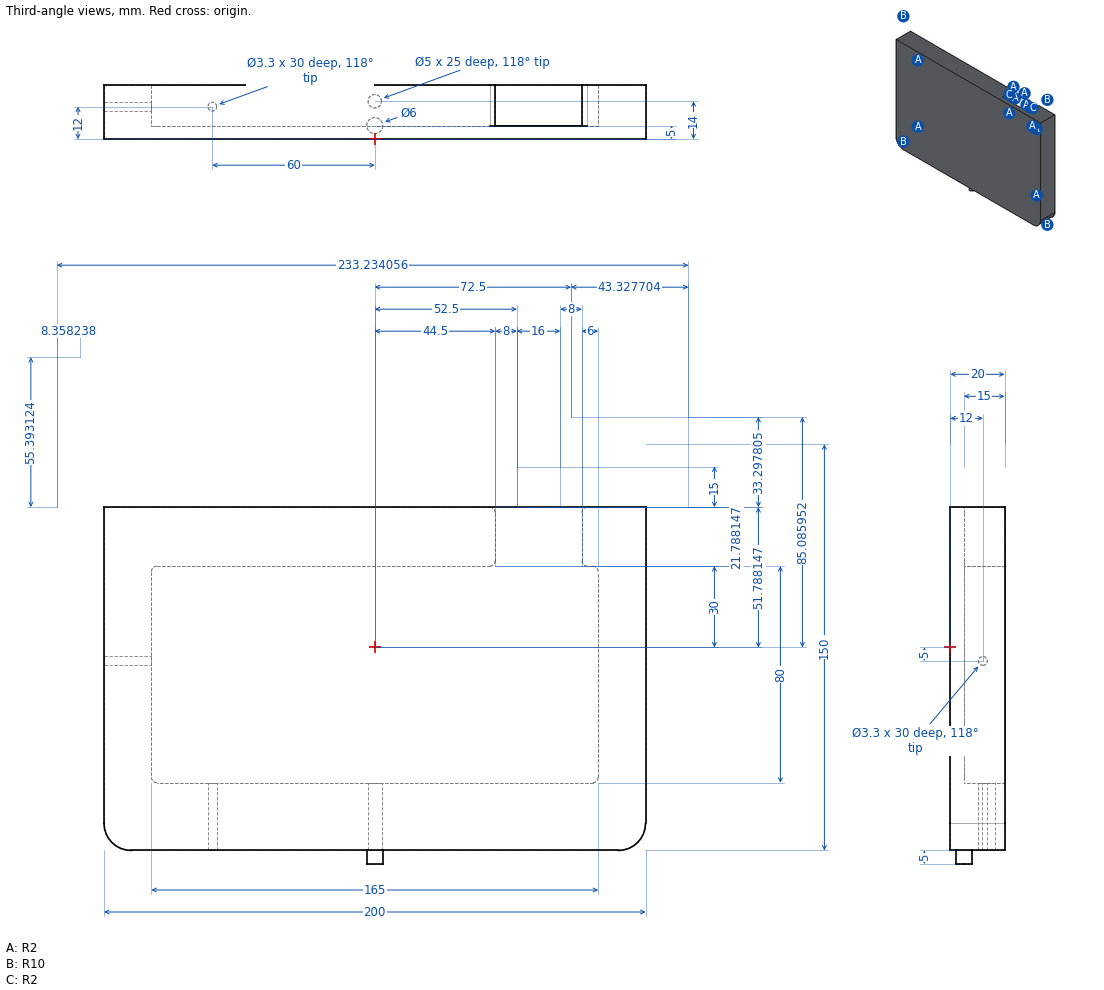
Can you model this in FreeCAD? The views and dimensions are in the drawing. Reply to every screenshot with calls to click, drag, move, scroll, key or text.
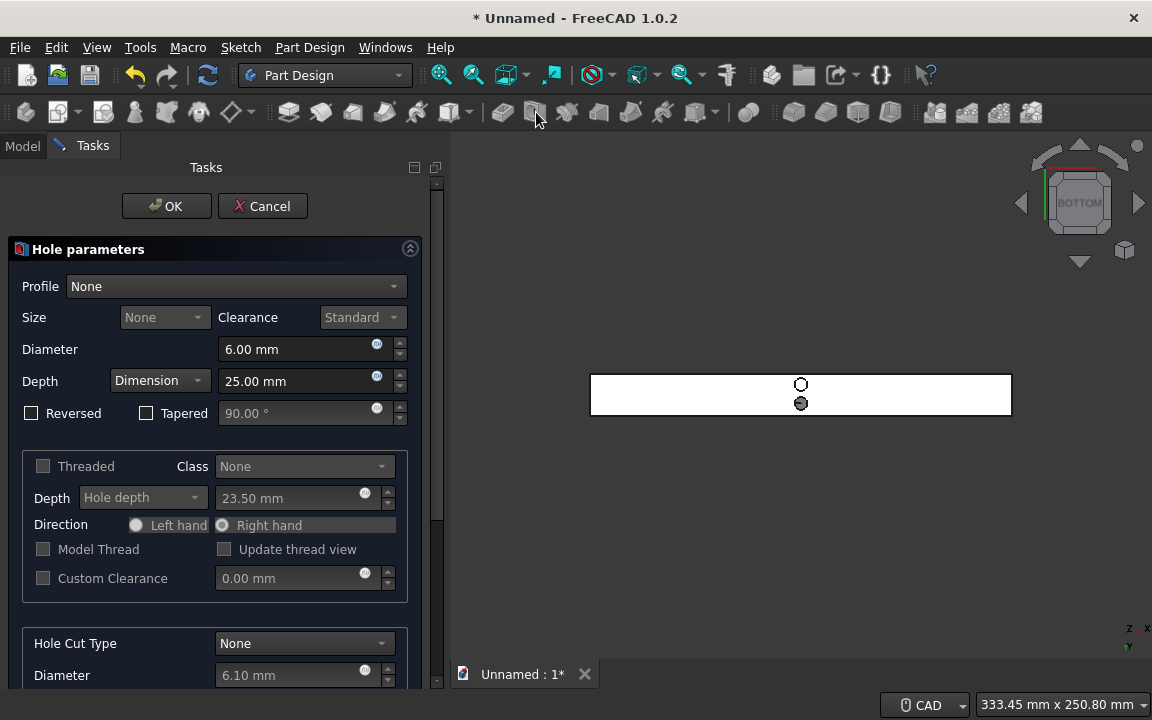
triple_click(305, 349)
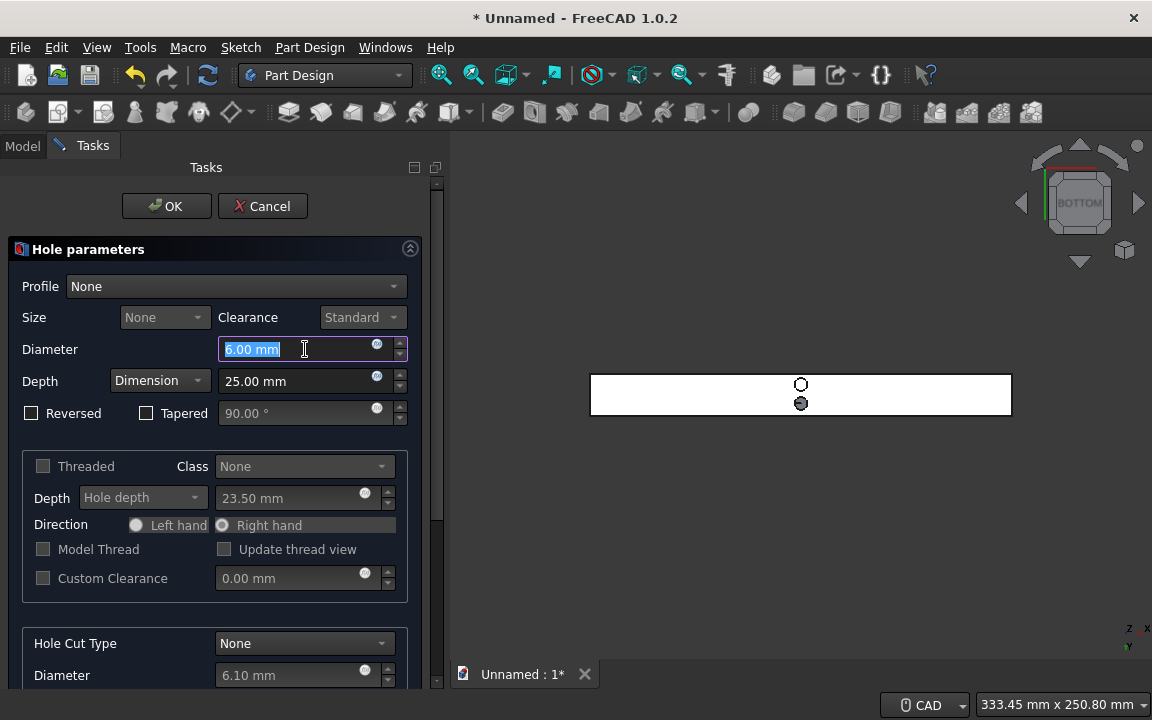
text(5)
key(Tab)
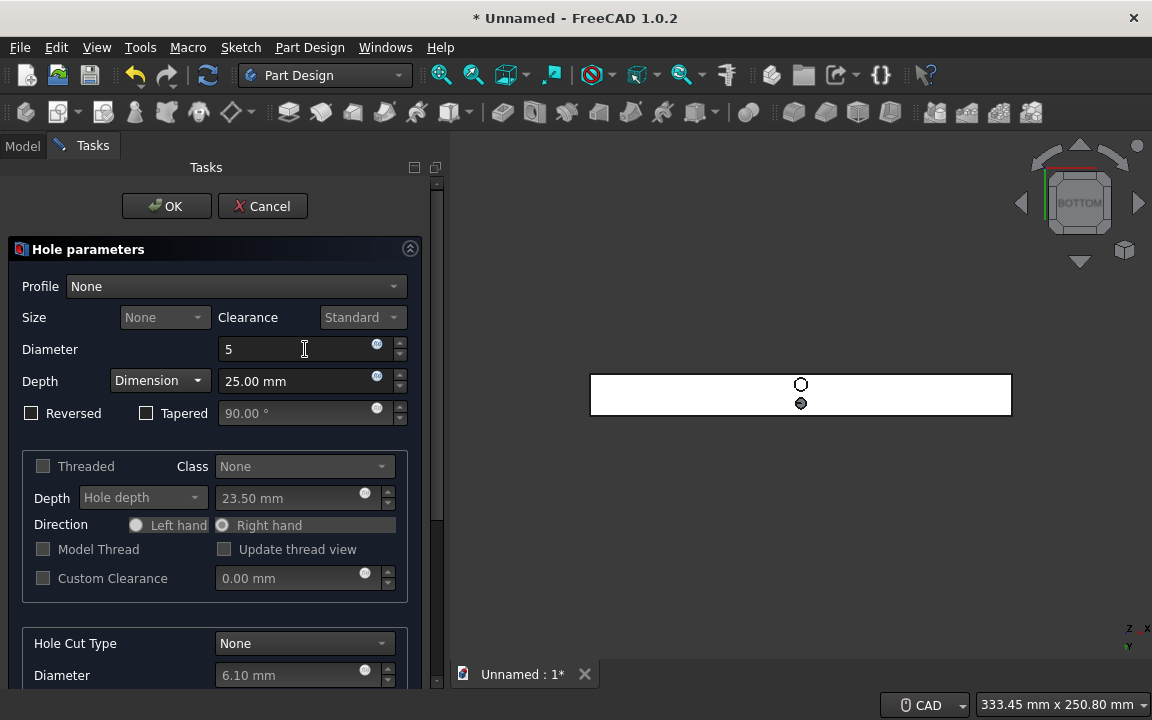
triple_click(305, 381)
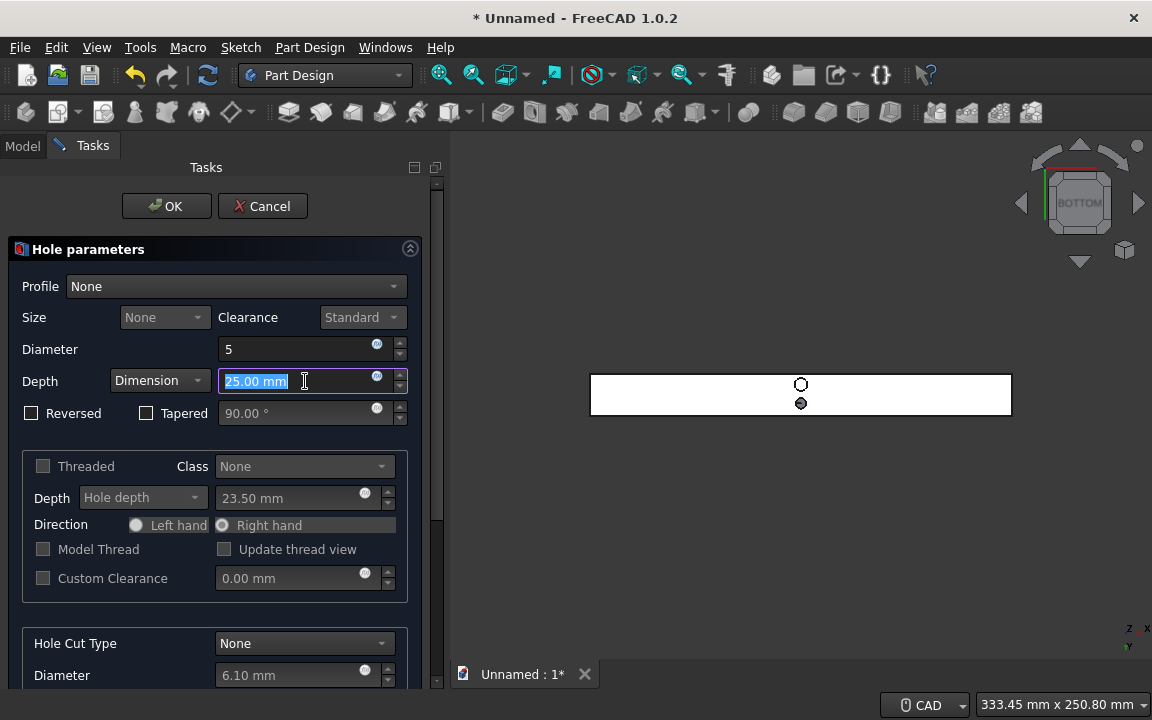
text(25)
key(Tab)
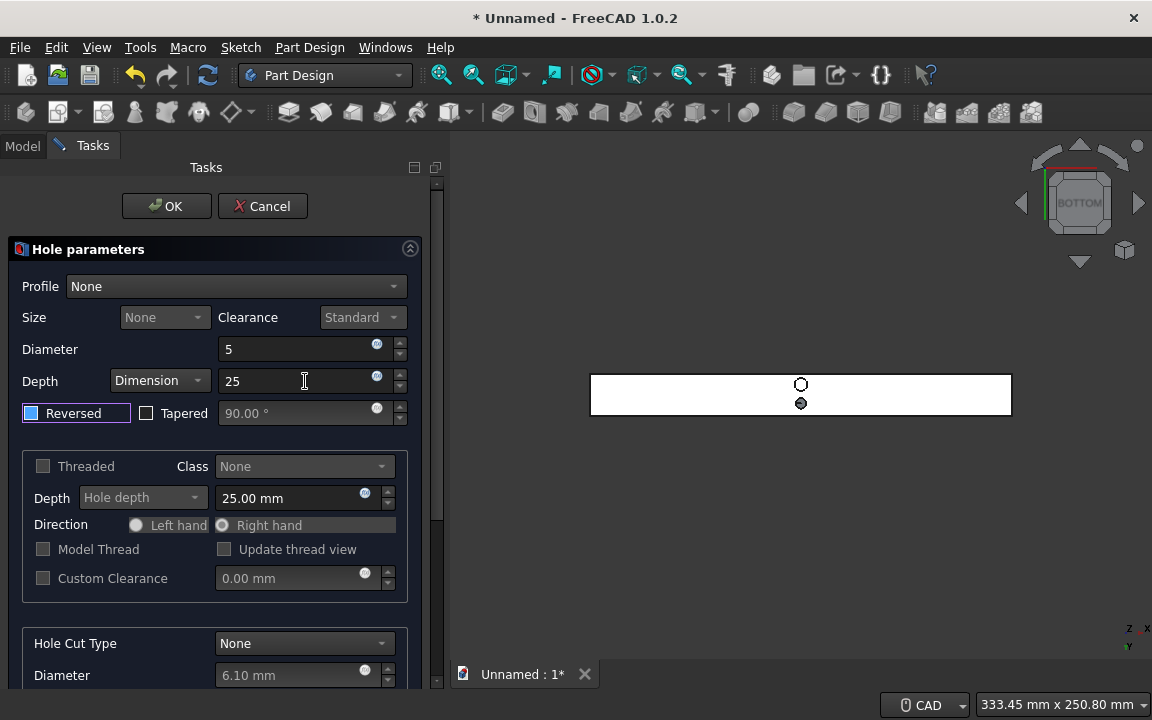
click(167, 206)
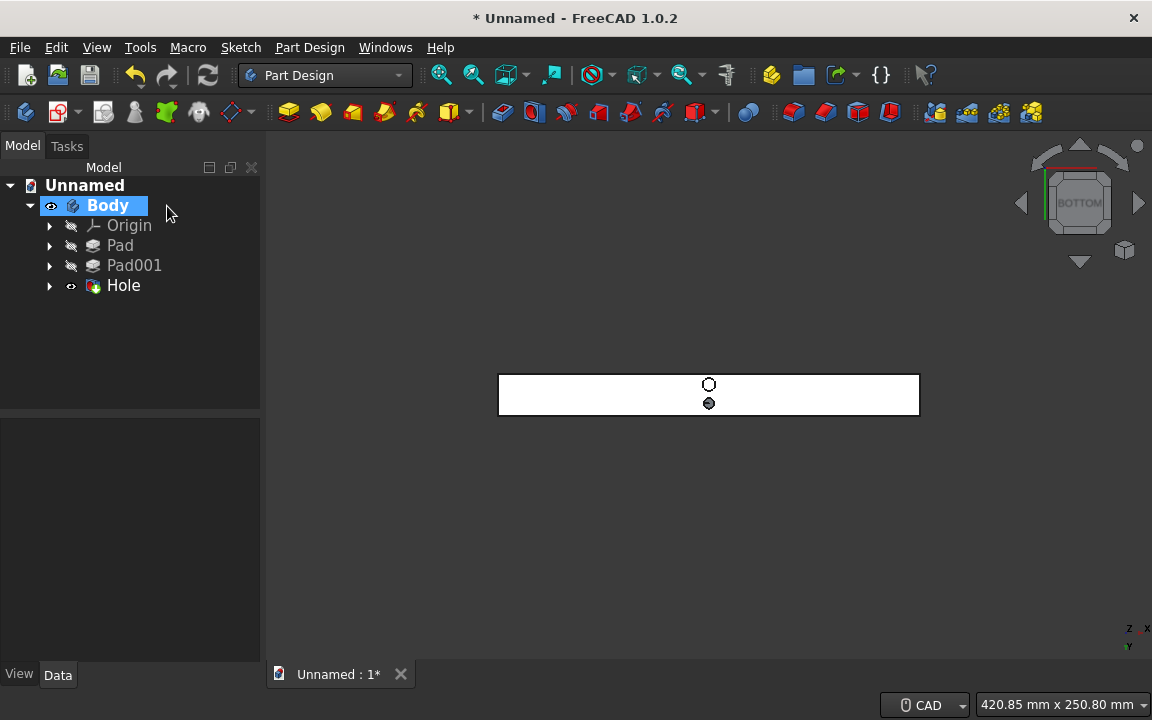
key(4)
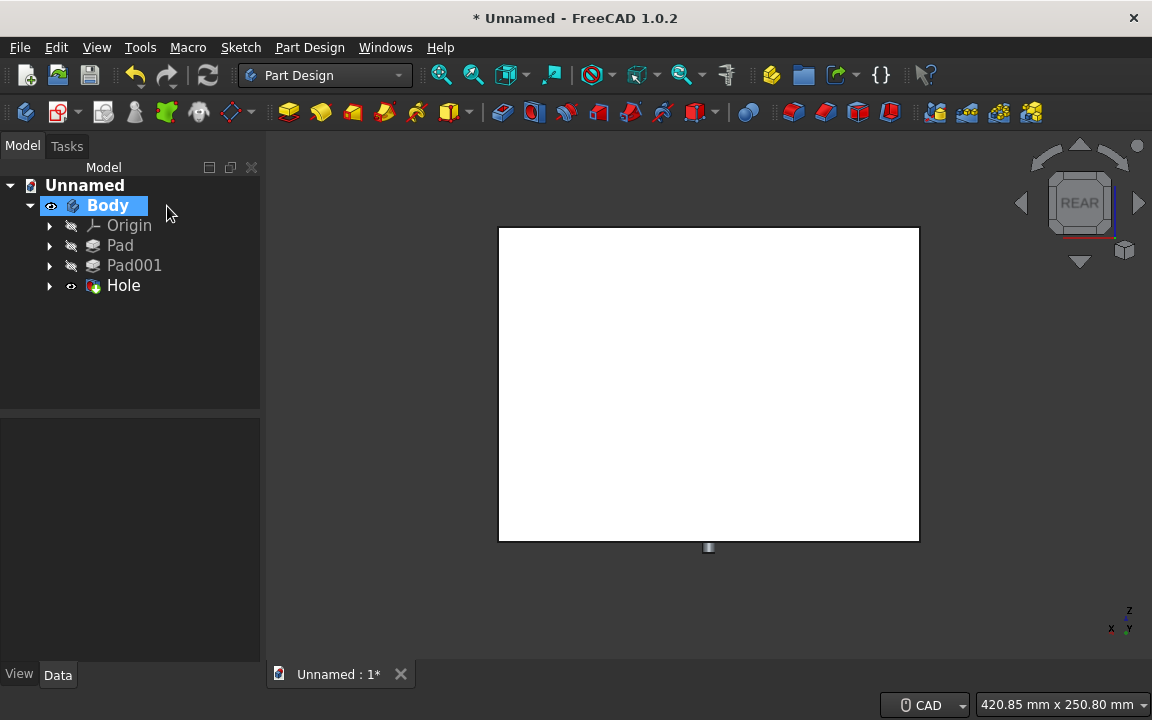
click(709, 383)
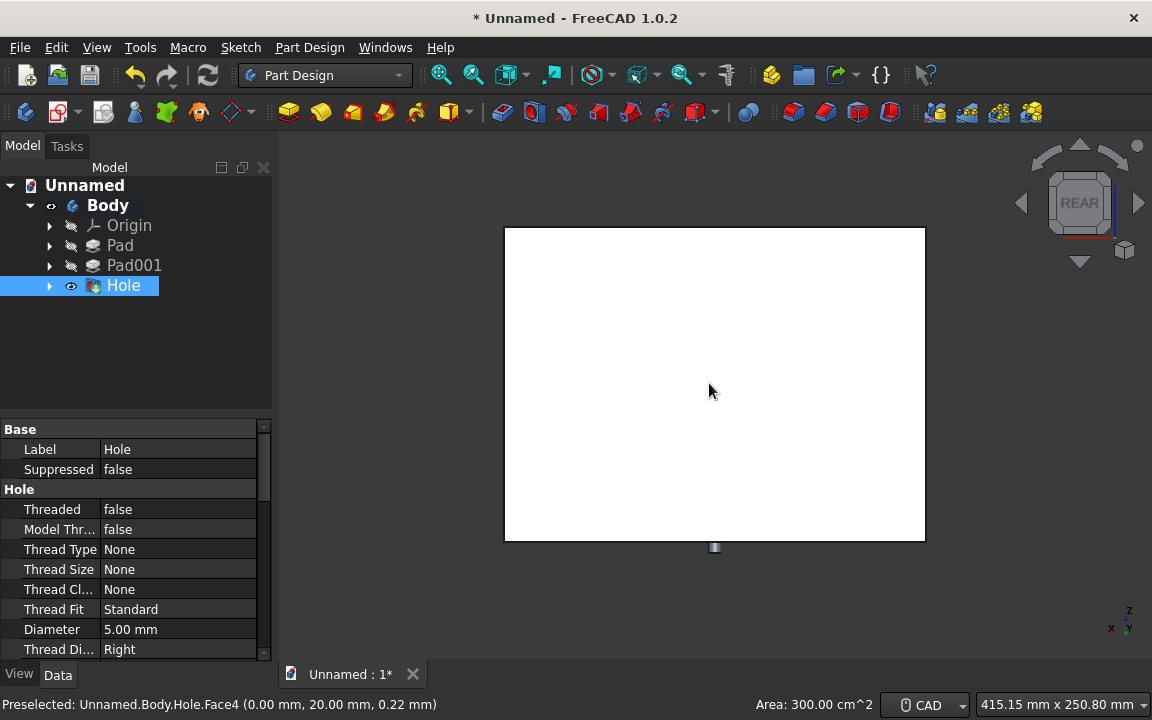
click(58, 112)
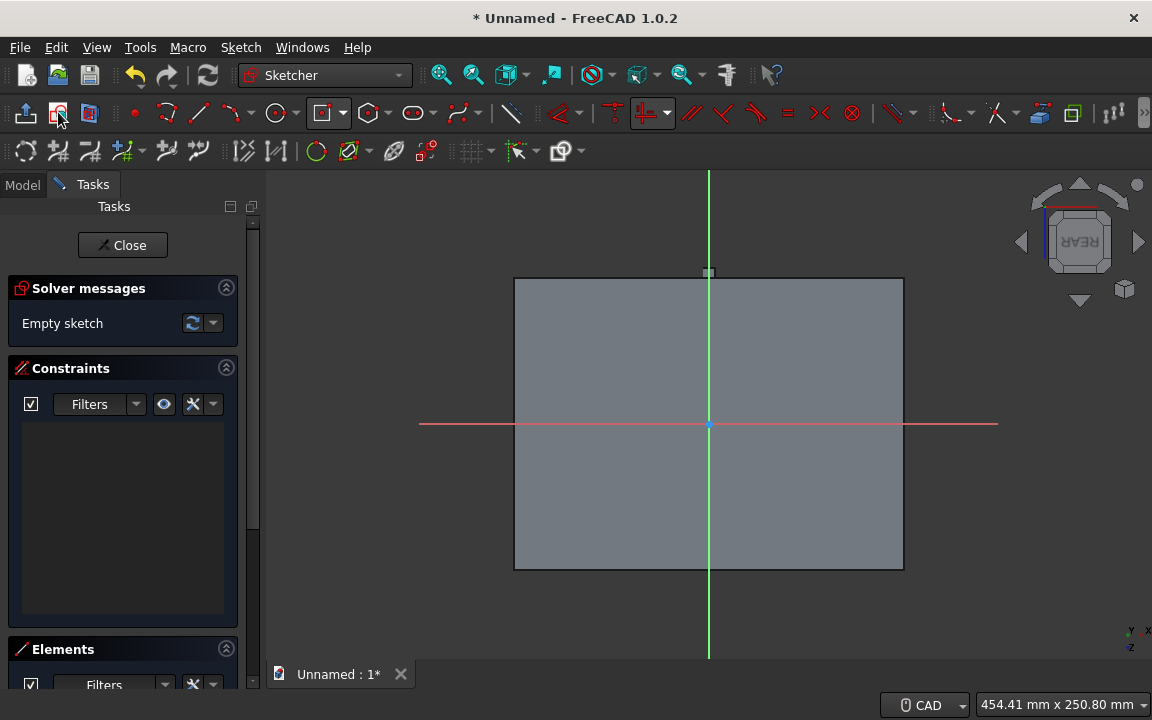
key(g)
key(m)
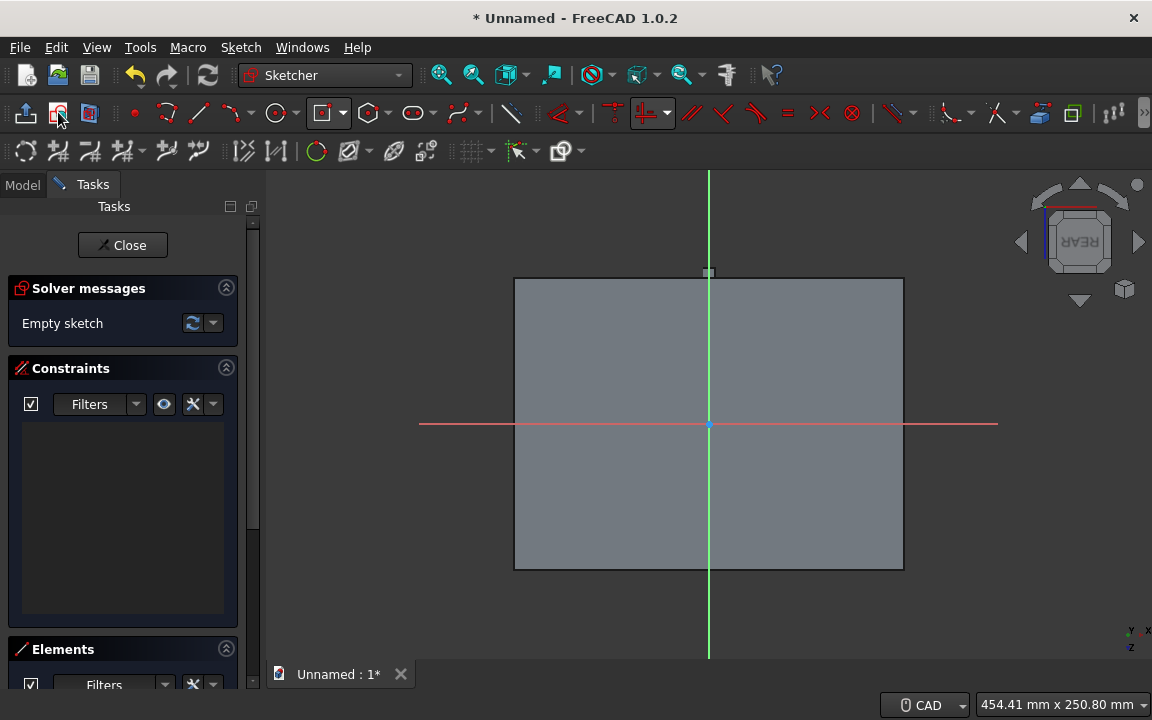
click(796, 483)
click(796, 525)
click(811, 525)
click(811, 554)
click(843, 554)
click(843, 525)
click(858, 525)
click(858, 483)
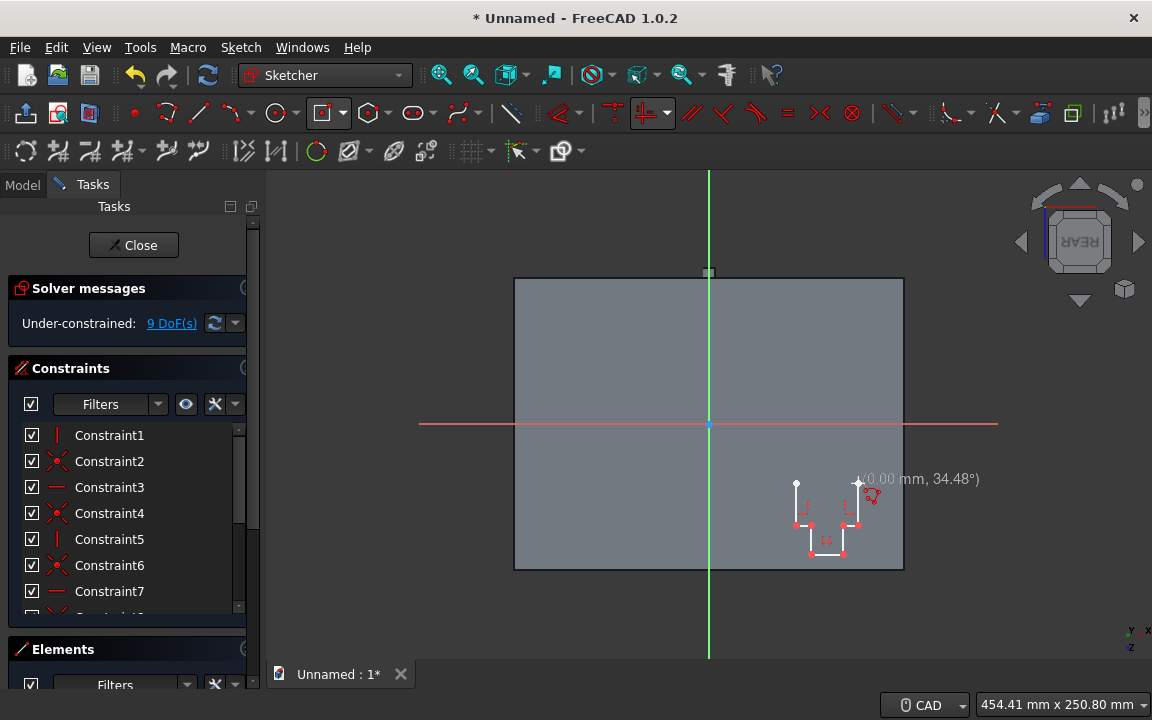
scroll(870, 483, up, 2)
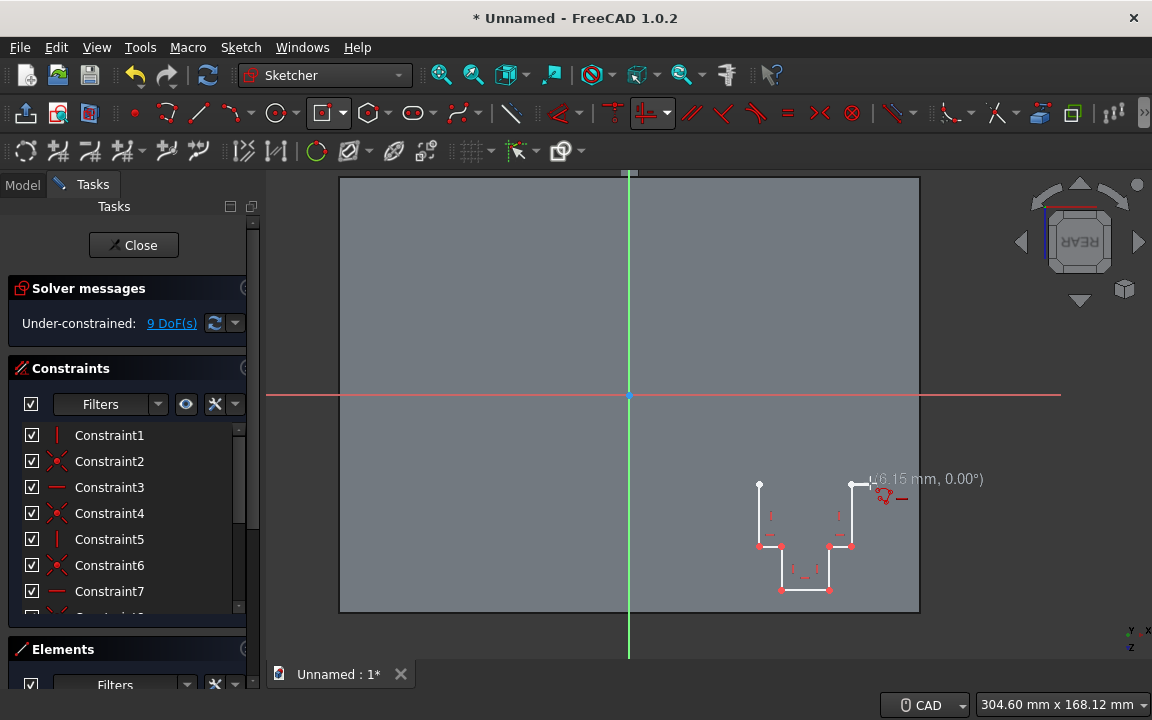
click(869, 483)
click(869, 250)
click(390, 250)
click(390, 482)
click(759, 484)
key(Escape)
key(Escape)